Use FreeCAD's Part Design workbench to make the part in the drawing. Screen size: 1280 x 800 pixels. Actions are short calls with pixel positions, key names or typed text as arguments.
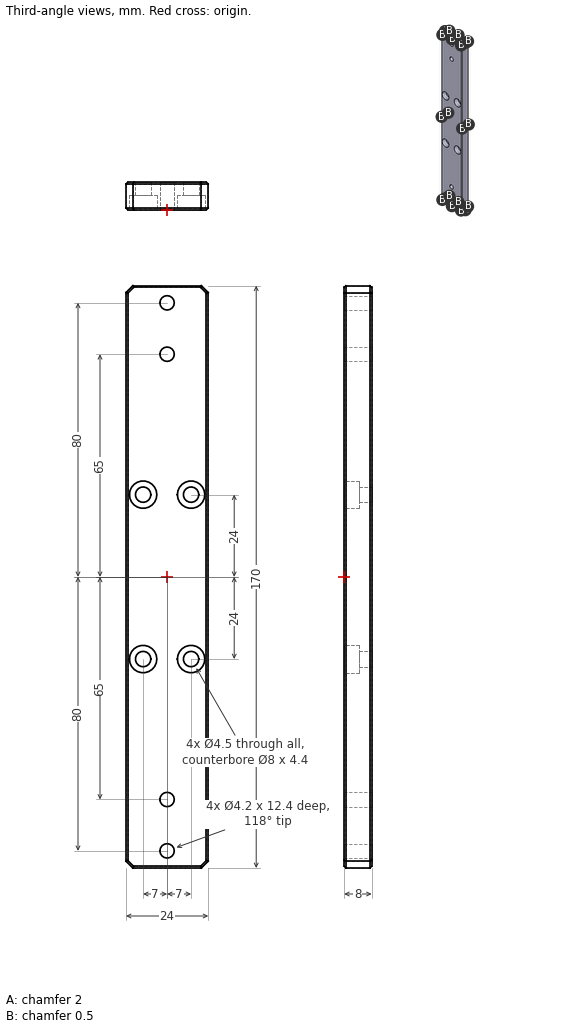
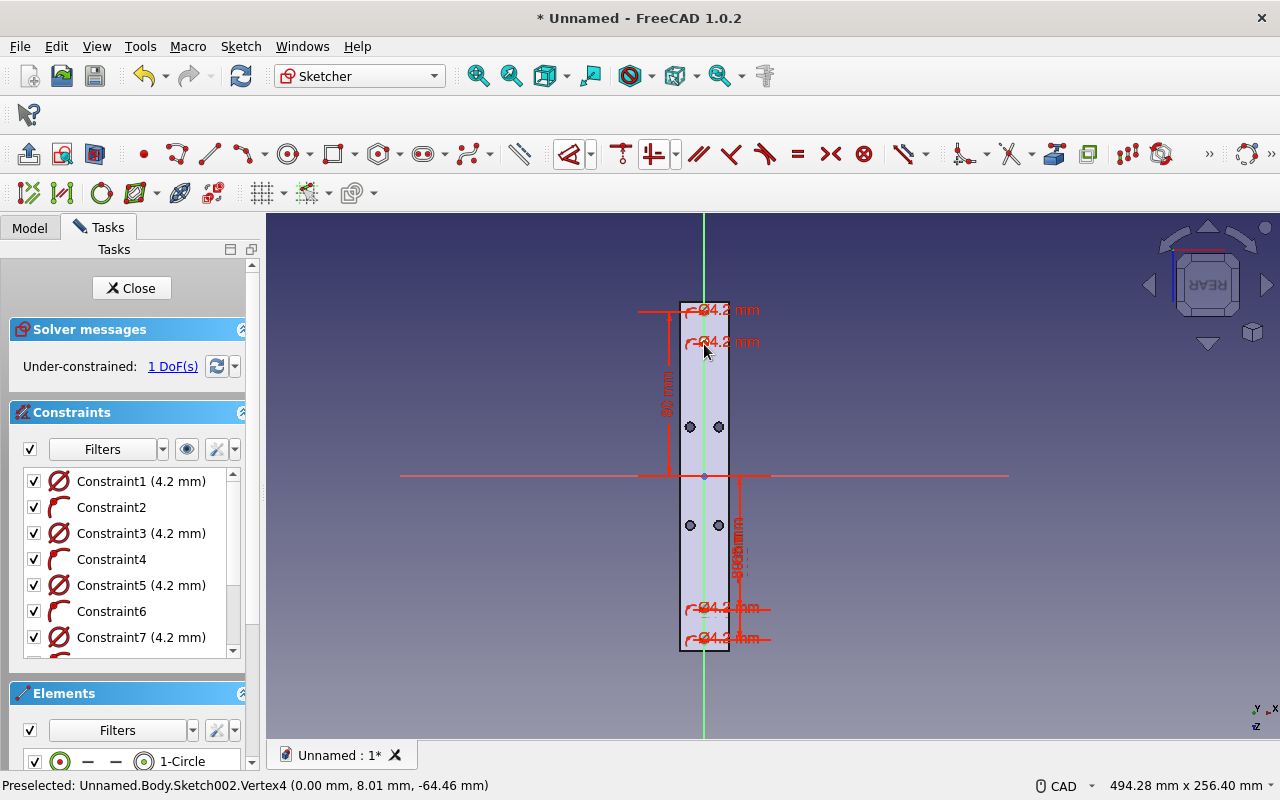
key(i)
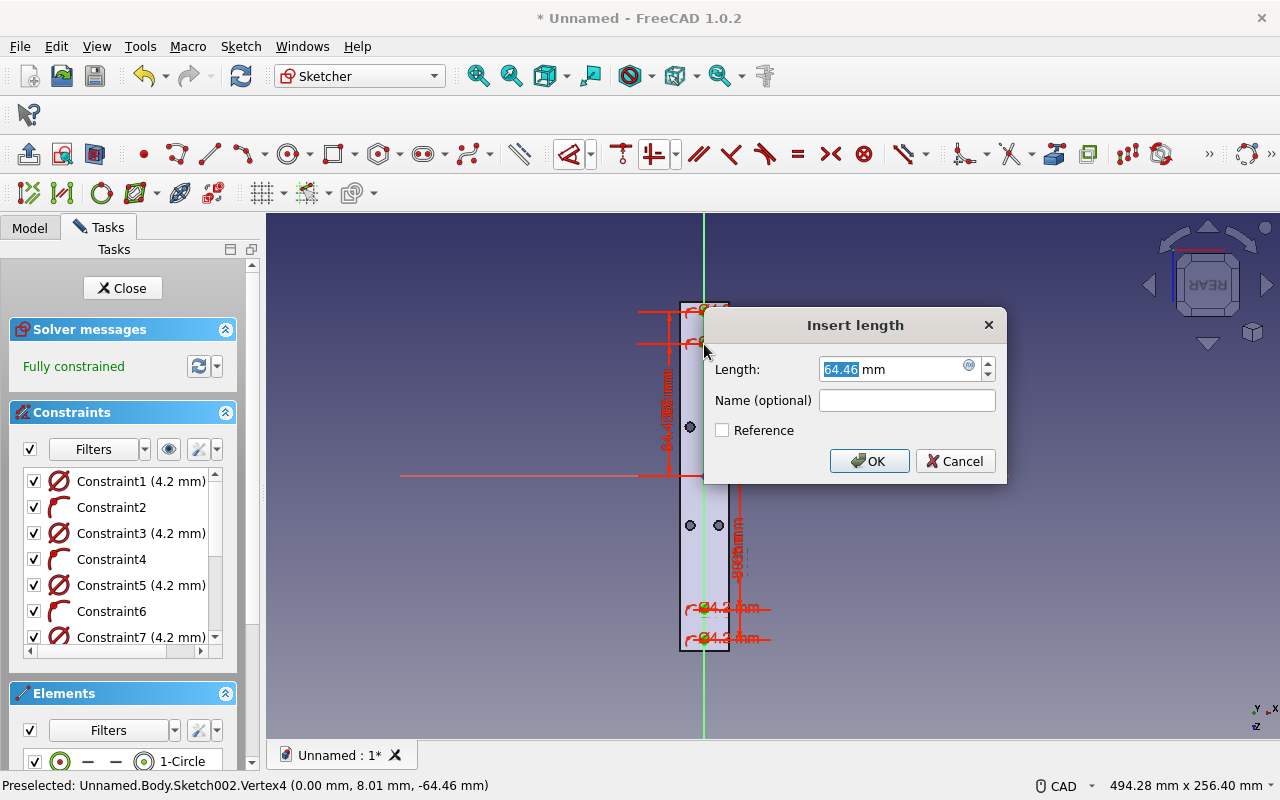
text(65)
key(Return)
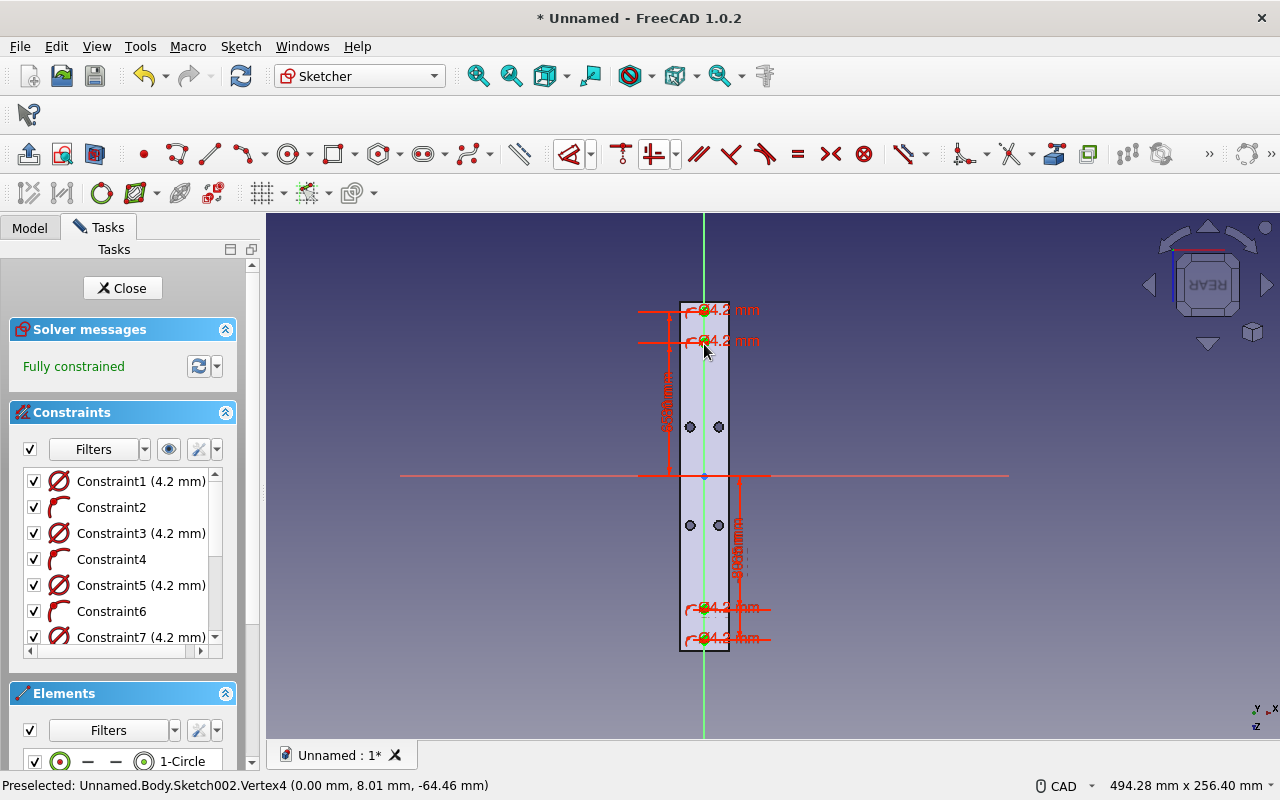
click(123, 288)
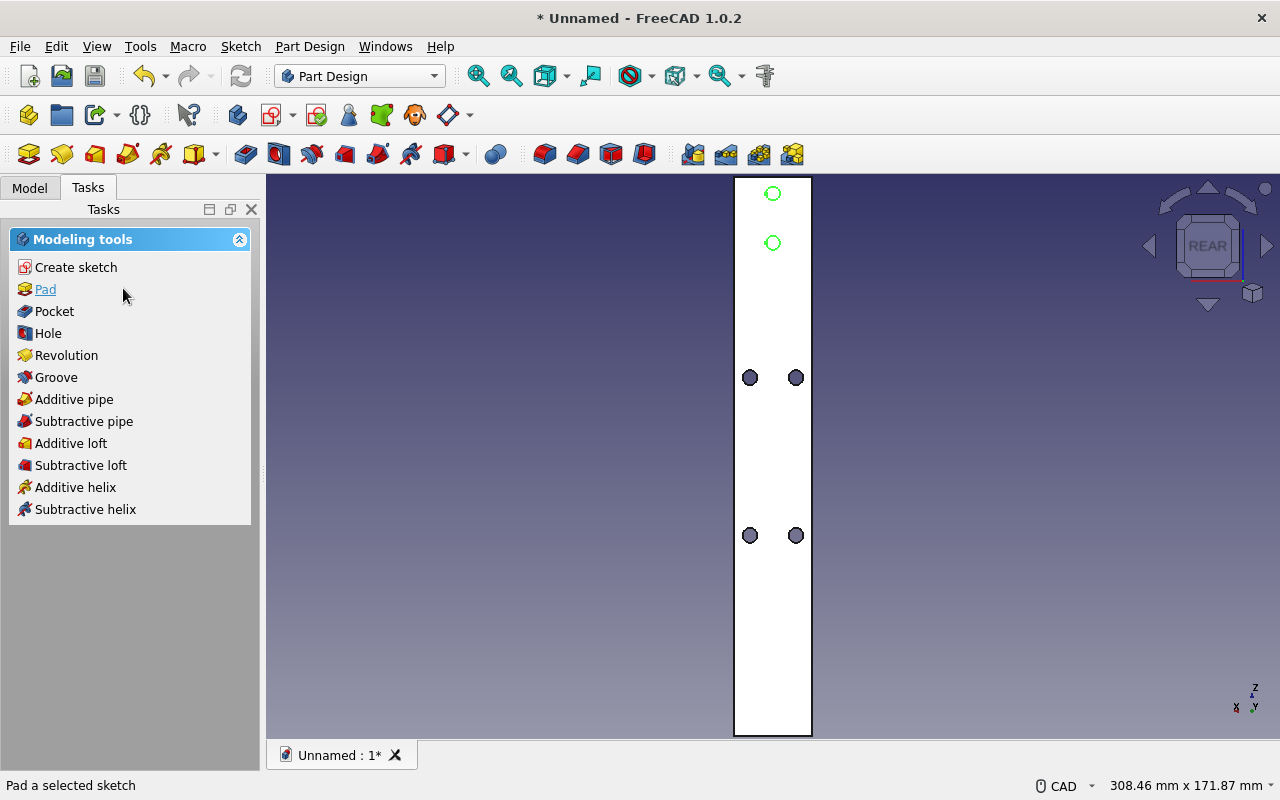
click(279, 154)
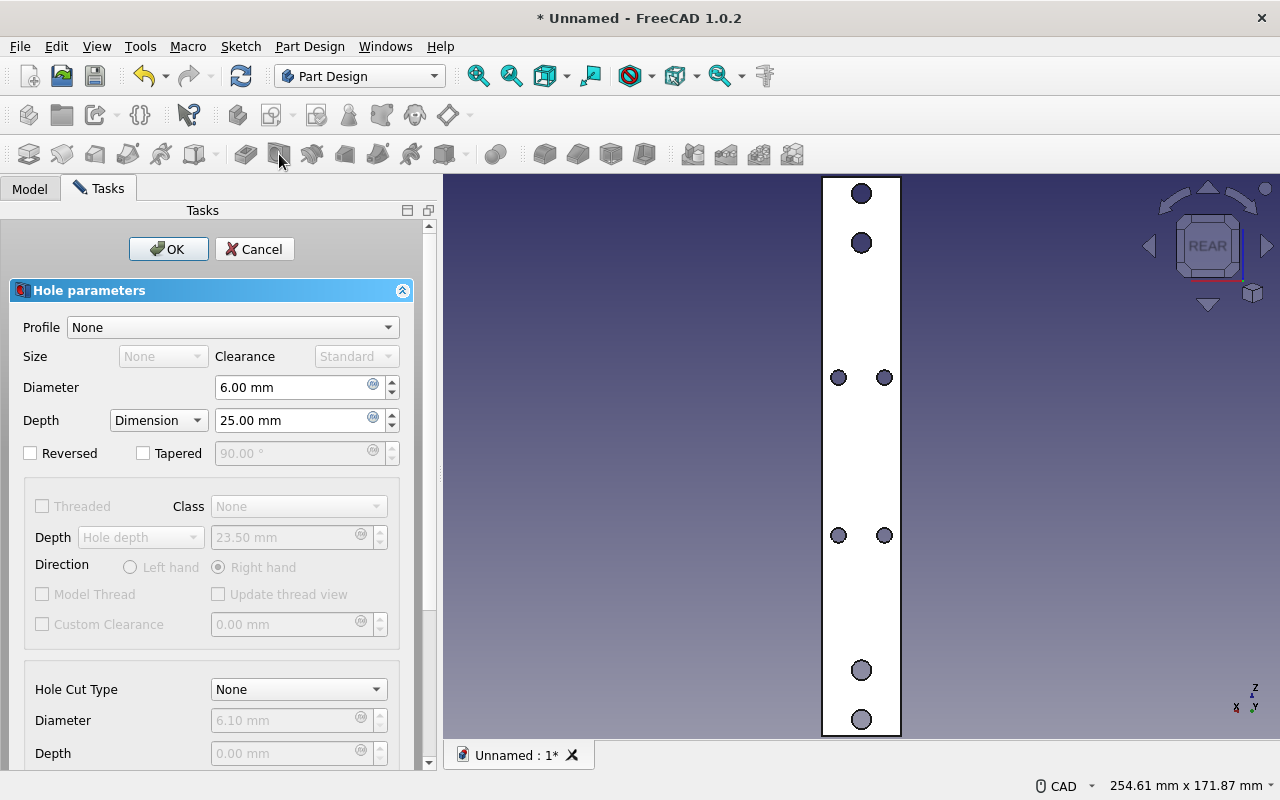
triple_click(300, 388)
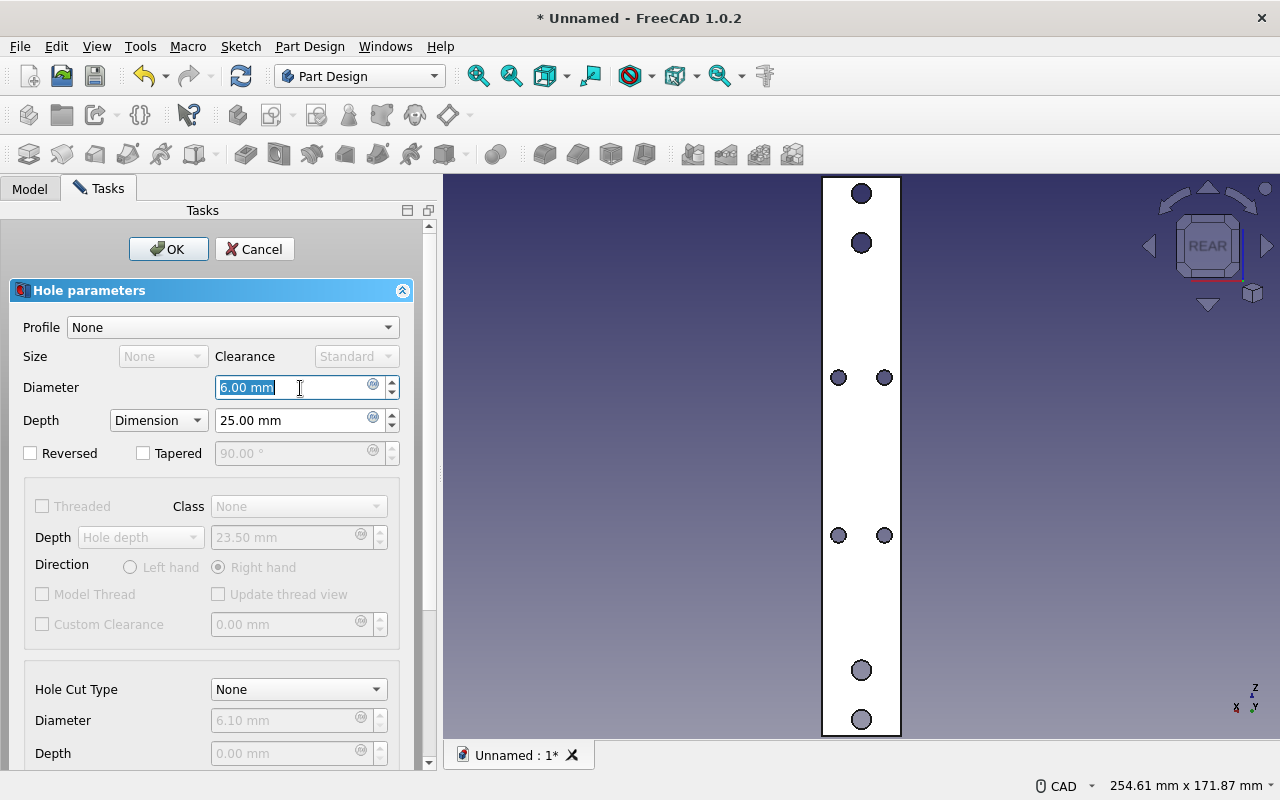
text(4.2)
key(Tab)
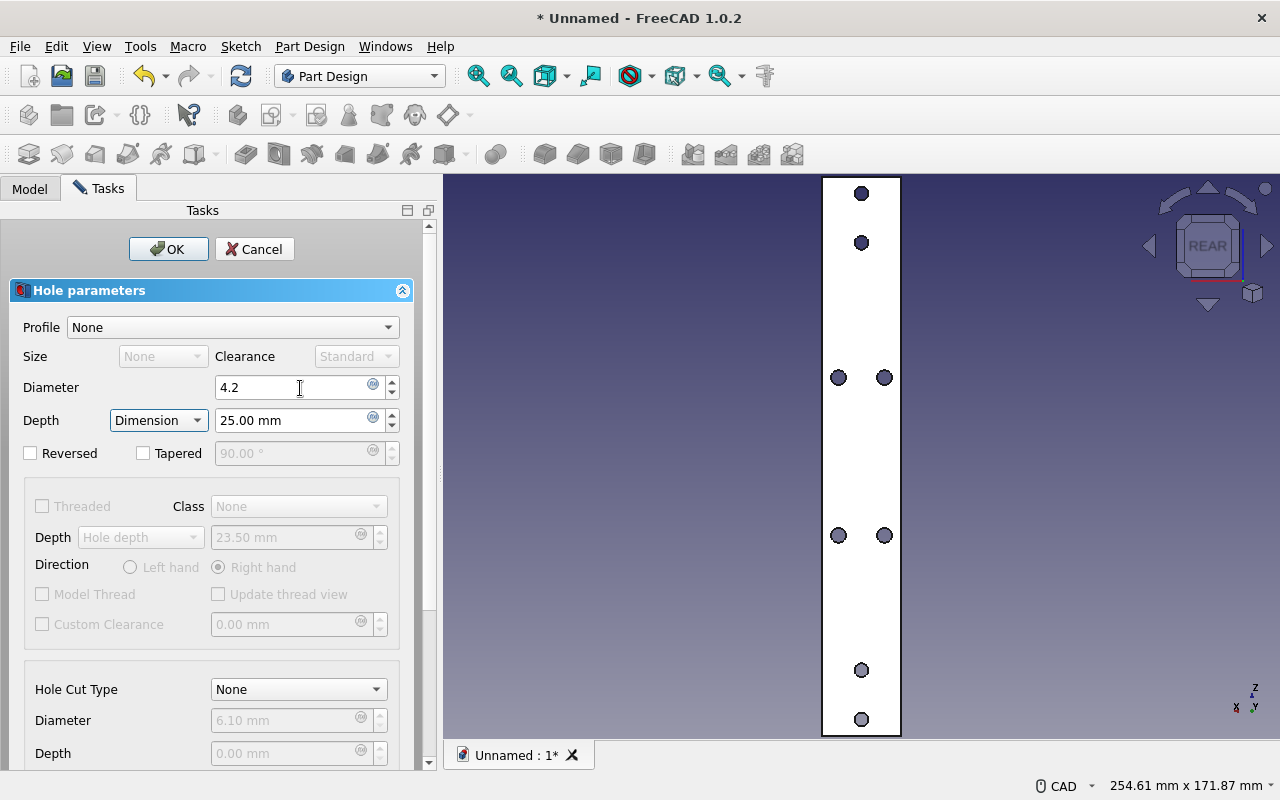
triple_click(300, 420)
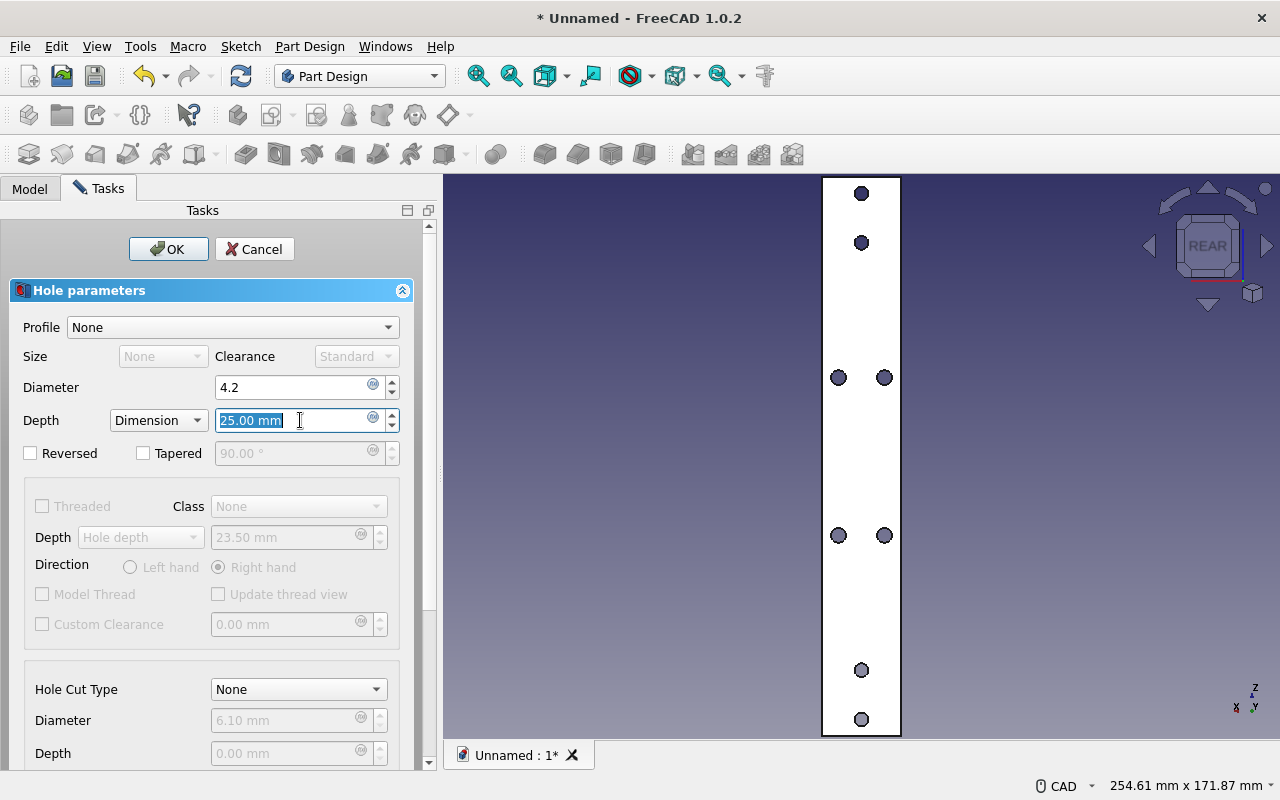
text(12.4)
key(Tab)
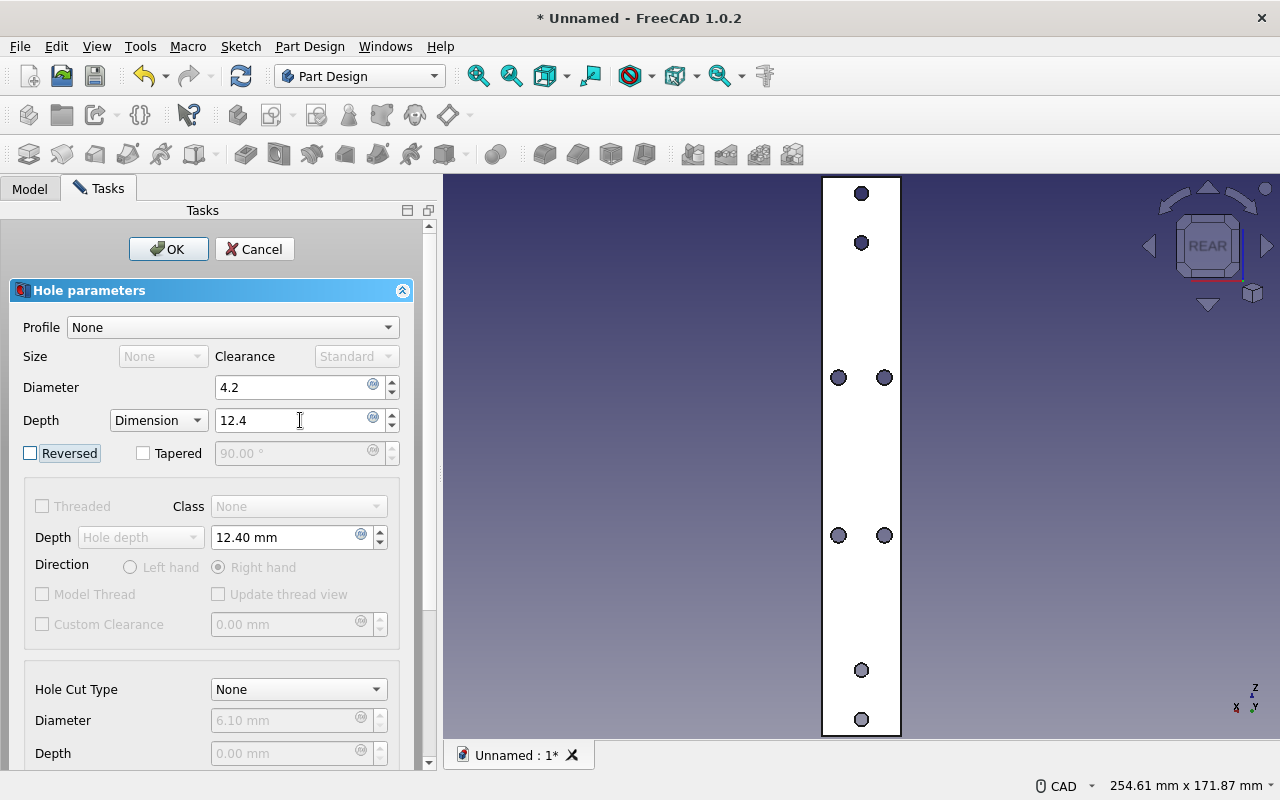
click(169, 249)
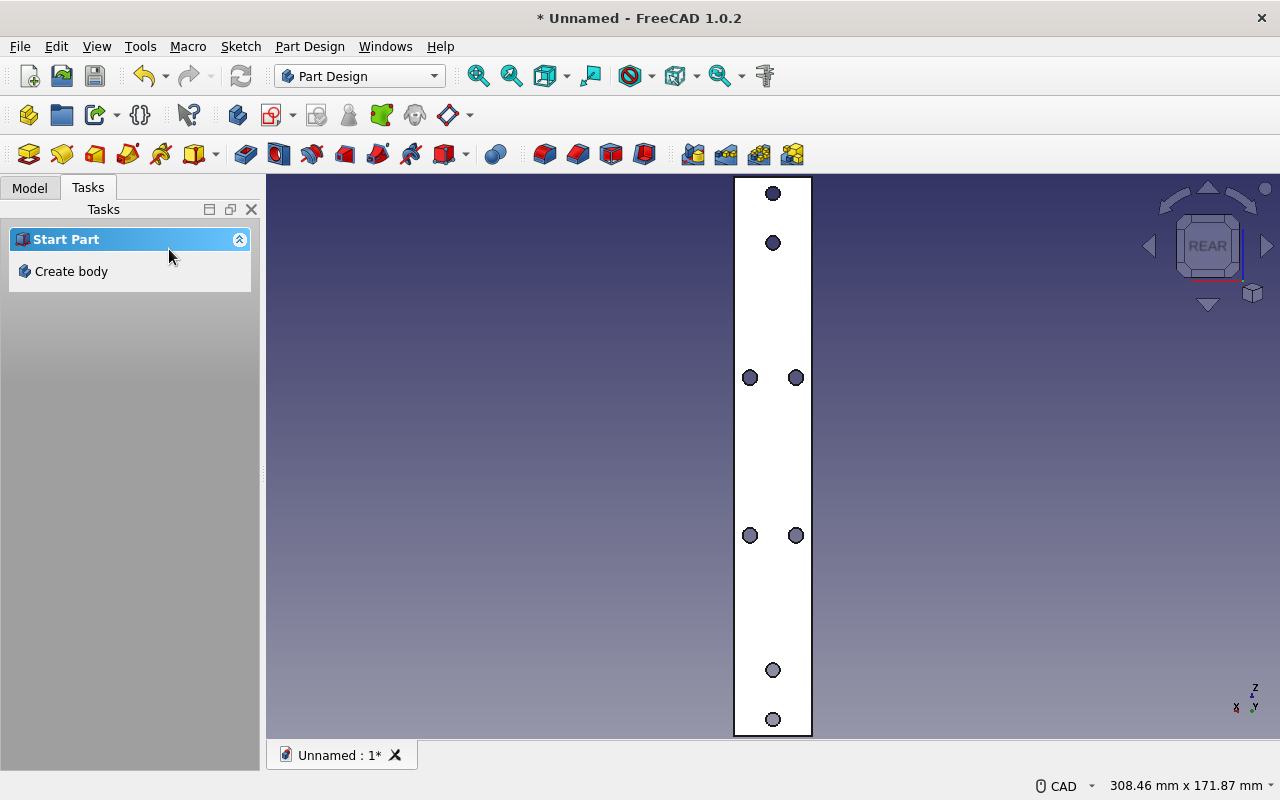
key(0)